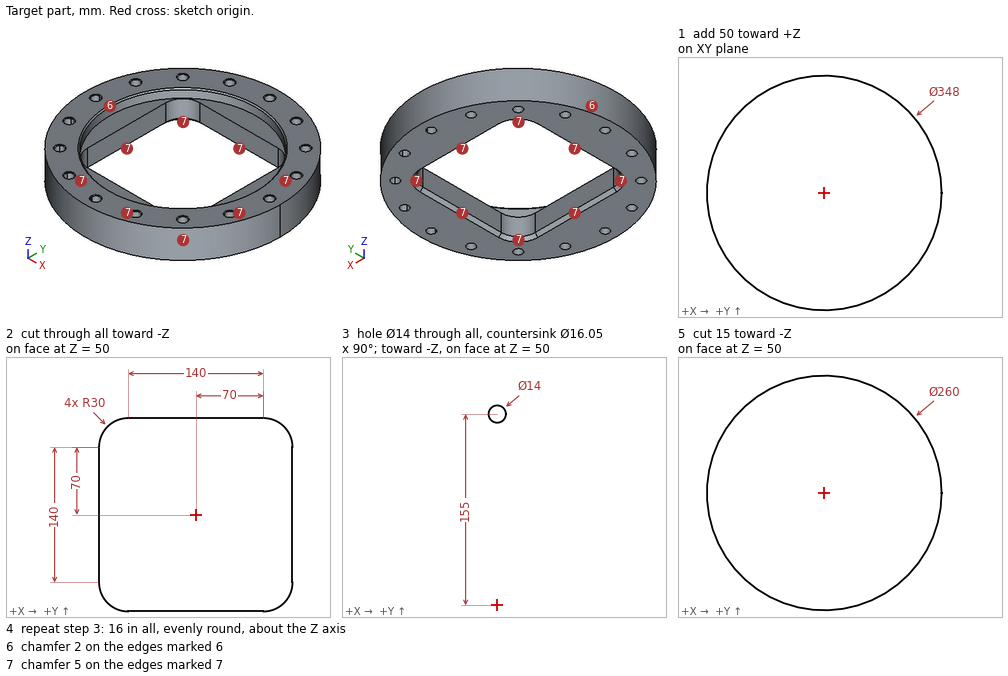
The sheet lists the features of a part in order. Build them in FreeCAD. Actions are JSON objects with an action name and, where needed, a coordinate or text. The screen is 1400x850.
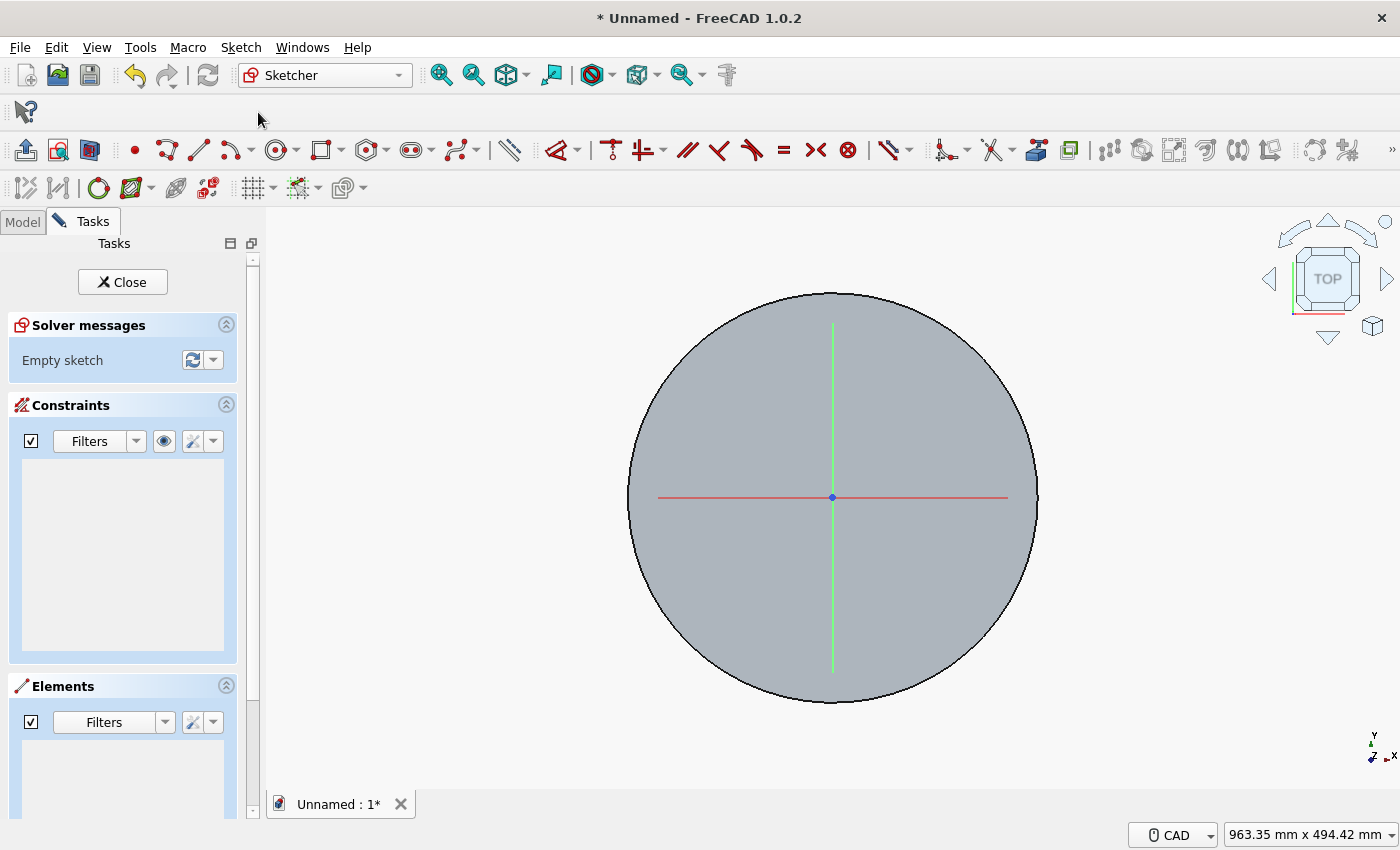
{"action": "scroll", "coordinate": [972, 498], "scroll_direction": "up", "scroll_amount": 2}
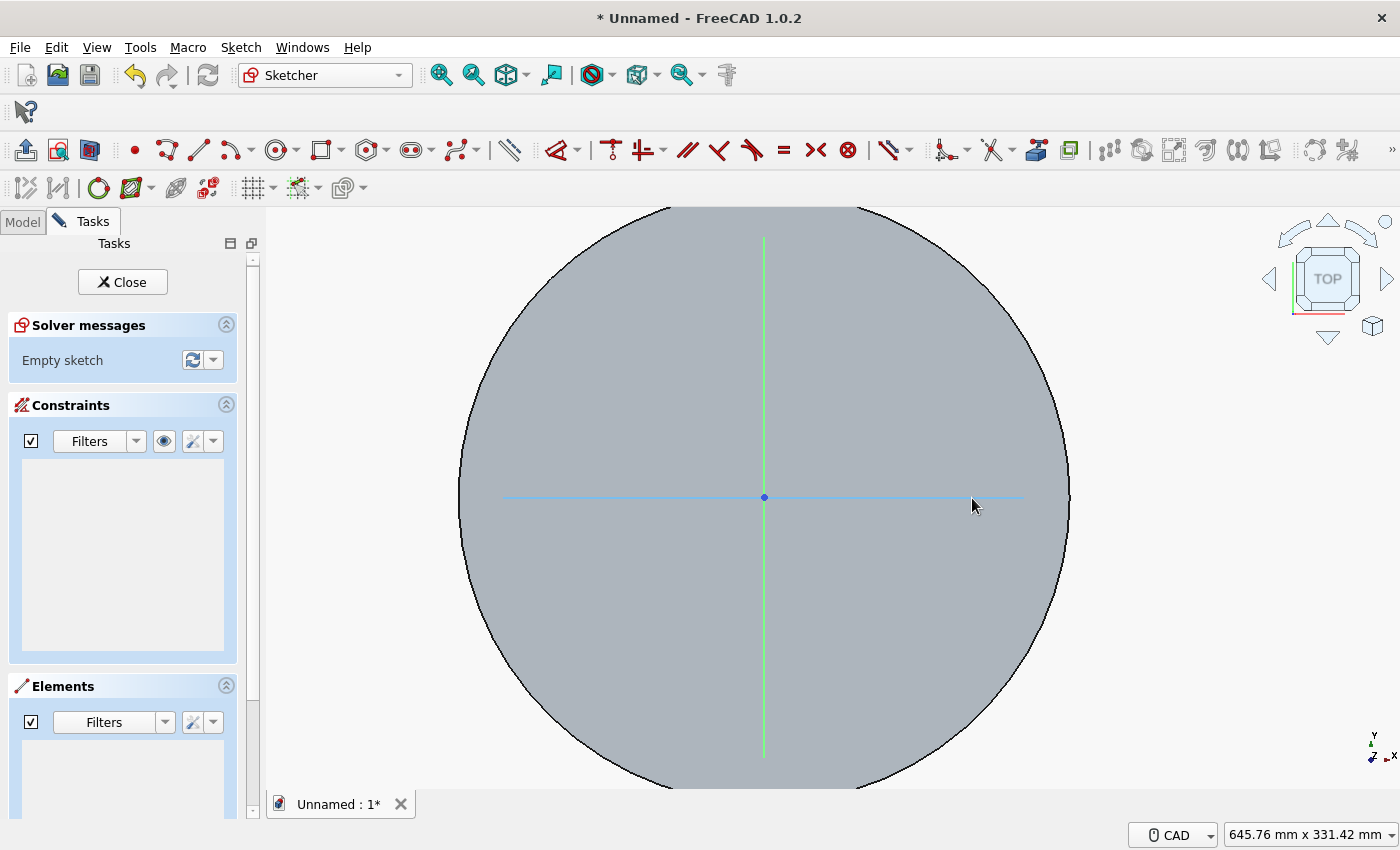
{"action": "left_click", "coordinate": [200, 150]}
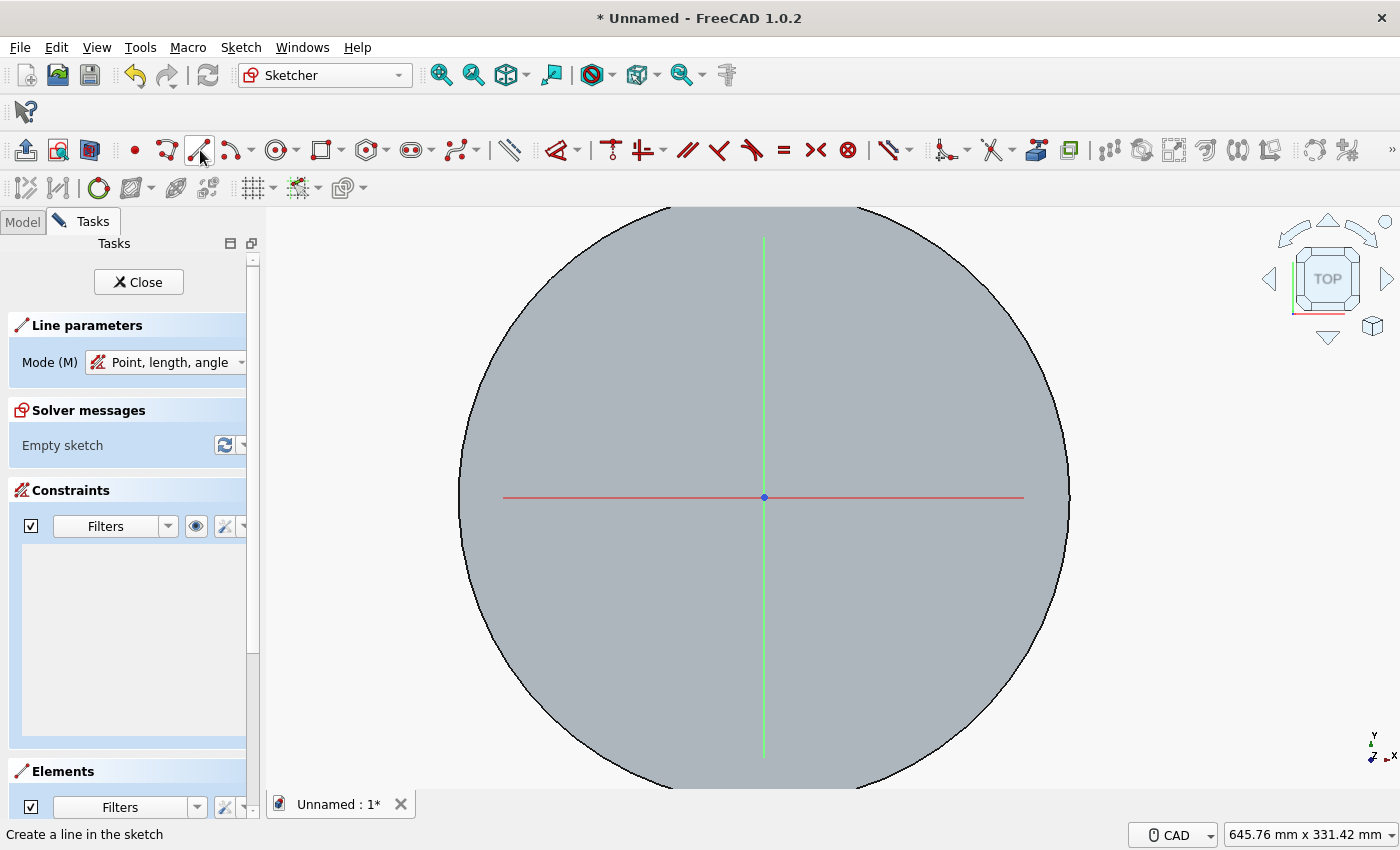
{"action": "left_click", "coordinate": [887, 322]}
{"action": "left_click", "coordinate": [641, 322]}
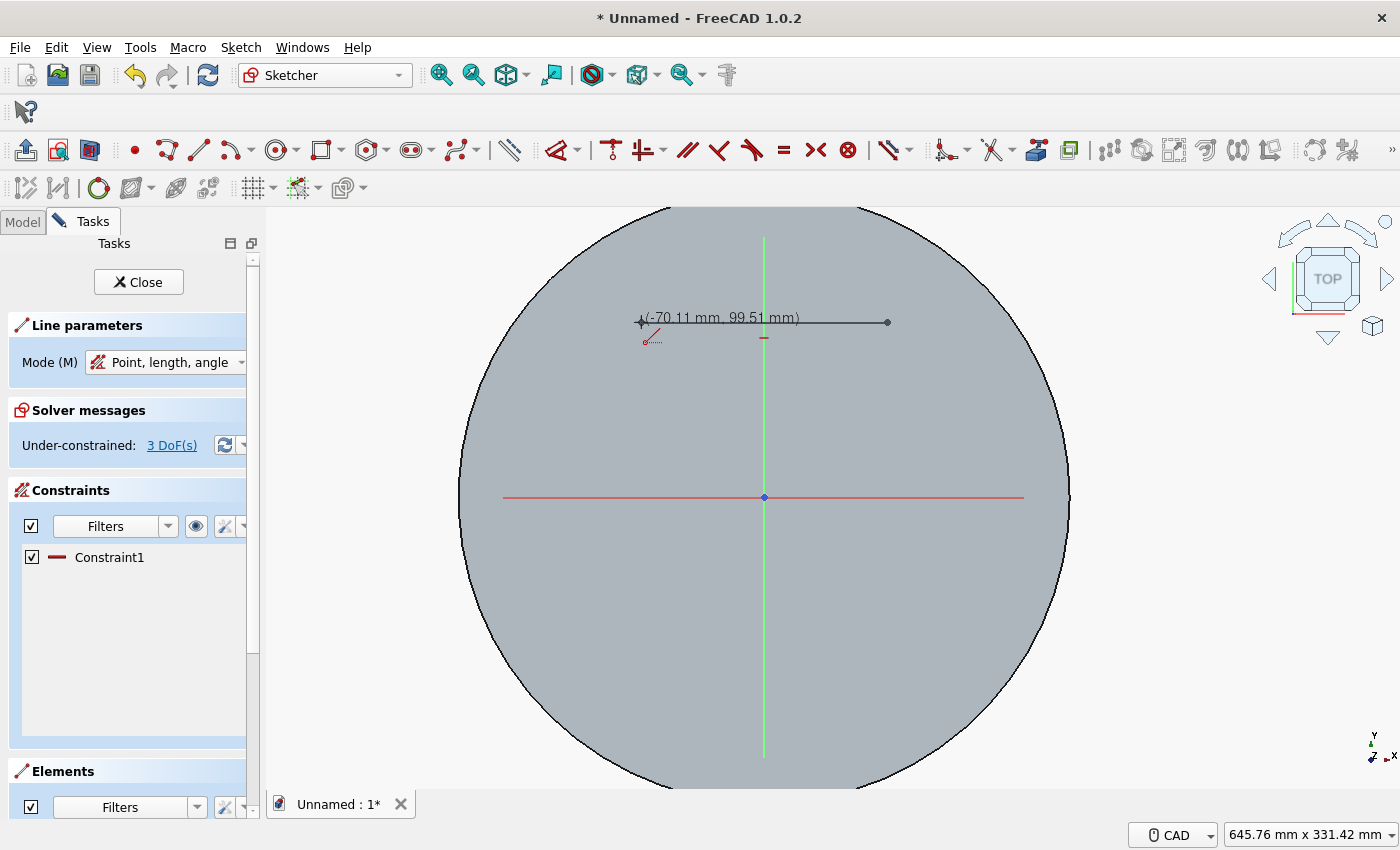
{"action": "left_click", "coordinate": [589, 375]}
{"action": "left_click", "coordinate": [589, 621]}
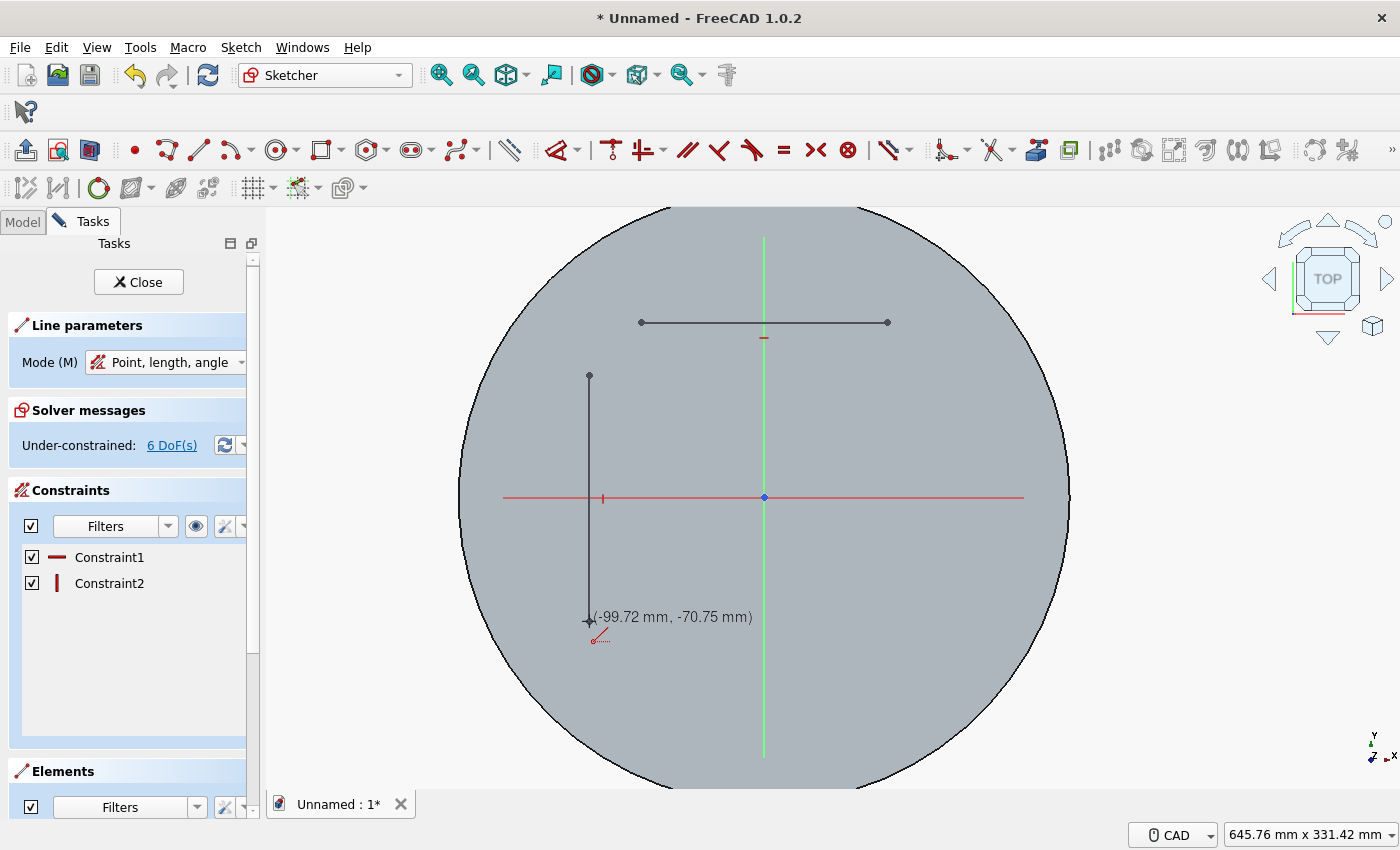
{"action": "left_click", "coordinate": [641, 673]}
{"action": "left_click", "coordinate": [887, 673]}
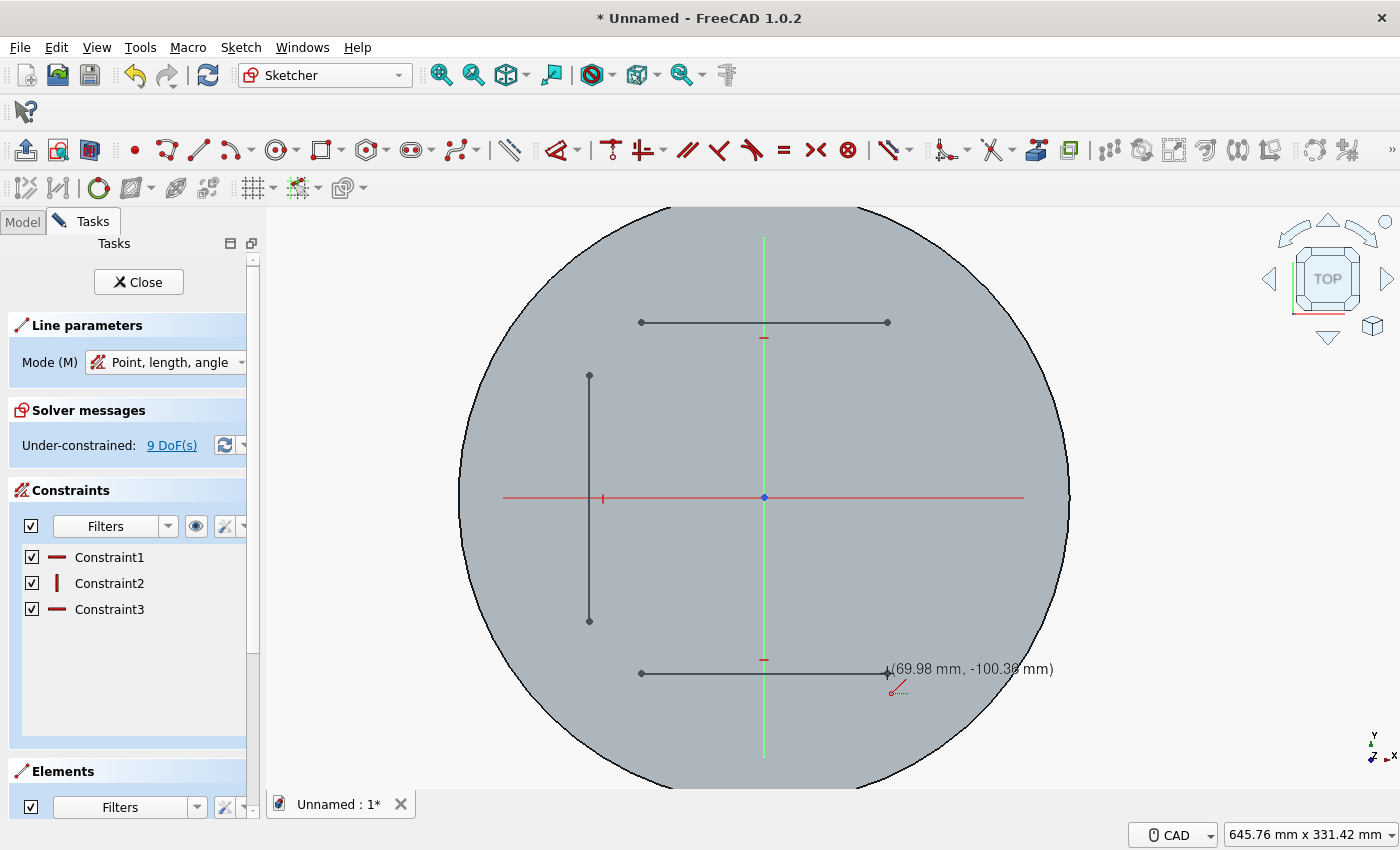
{"action": "left_click", "coordinate": [940, 621]}
{"action": "left_click", "coordinate": [940, 375]}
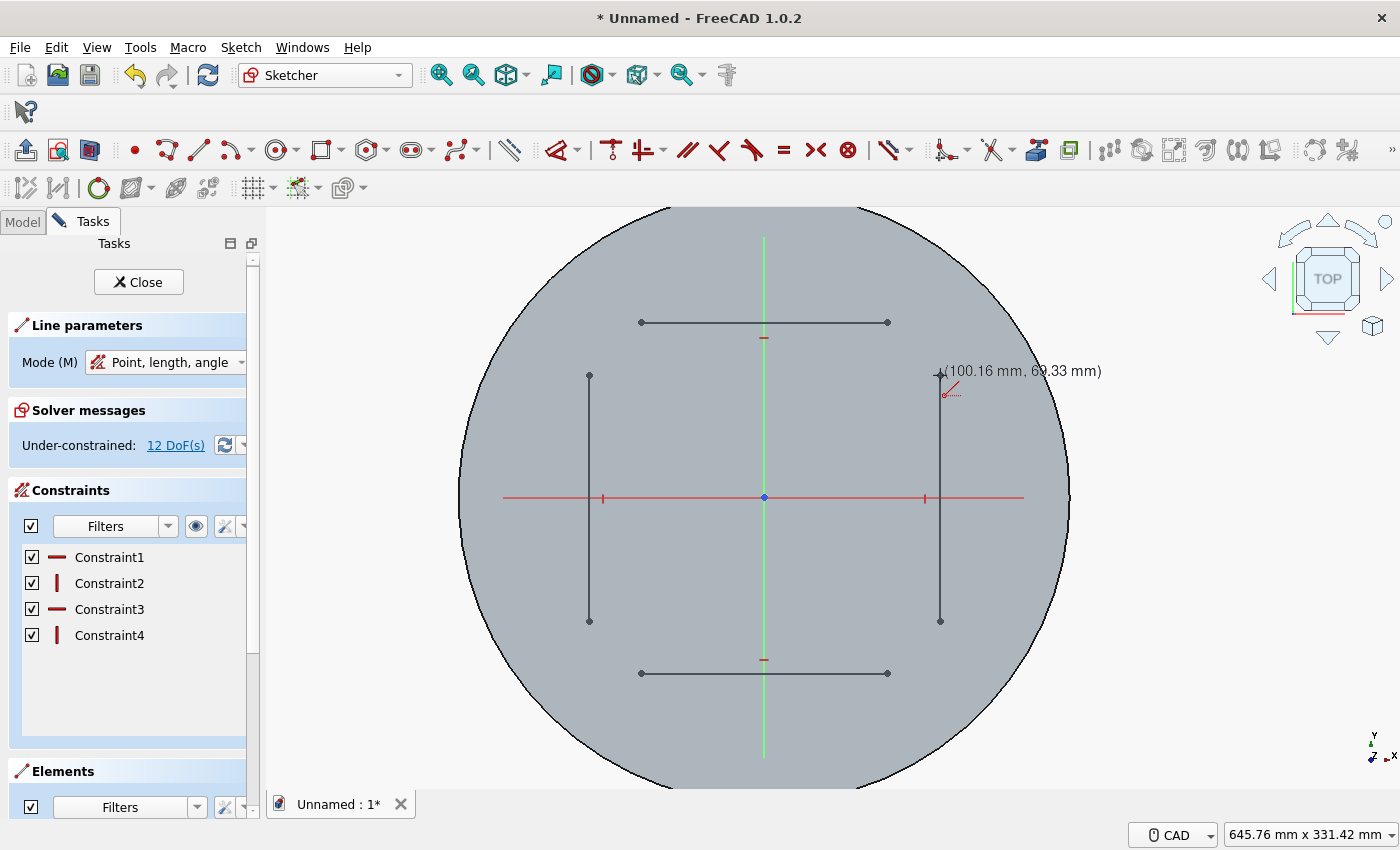
{"action": "left_click", "coordinate": [254, 150]}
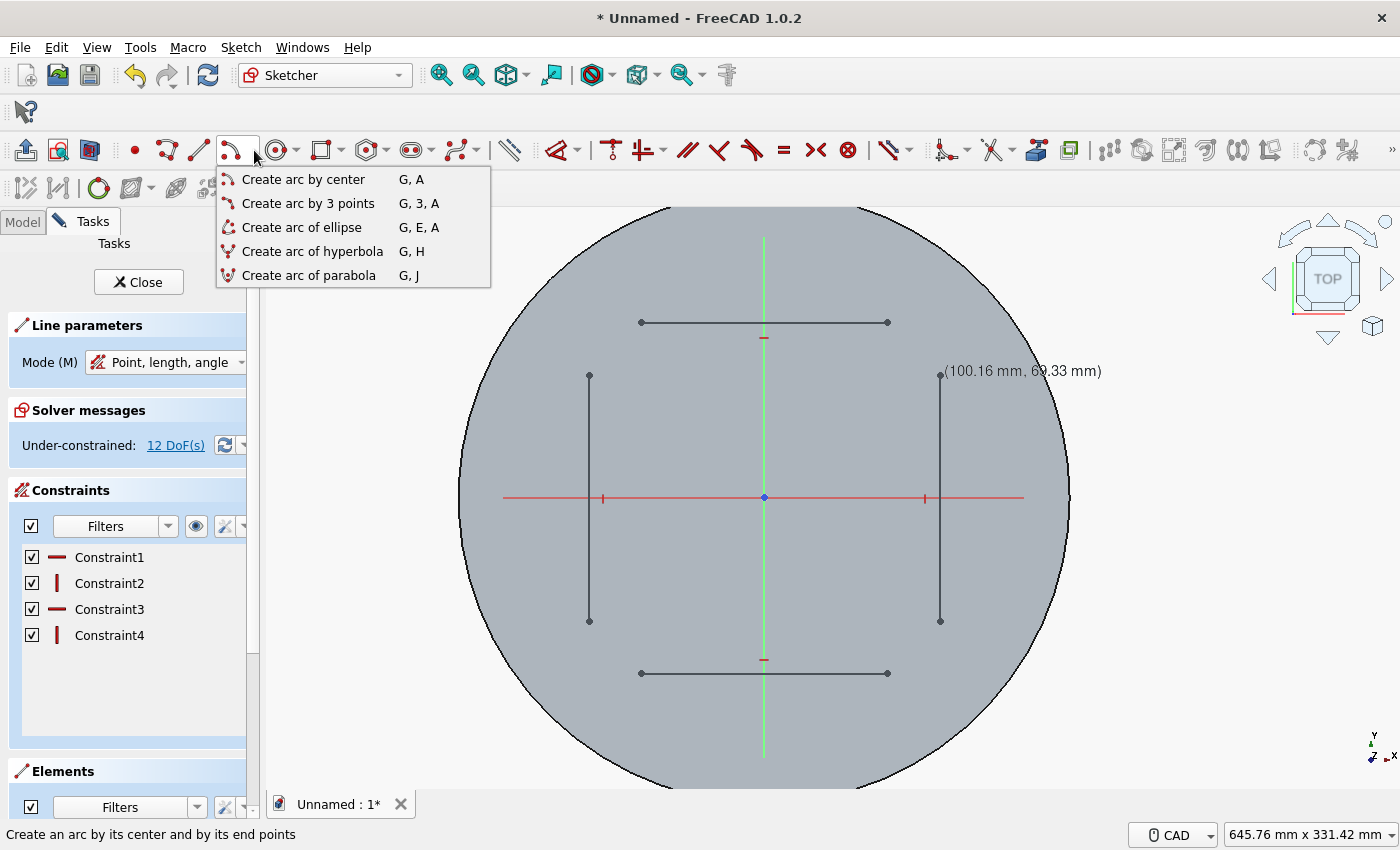
{"action": "left_click", "coordinate": [354, 203]}